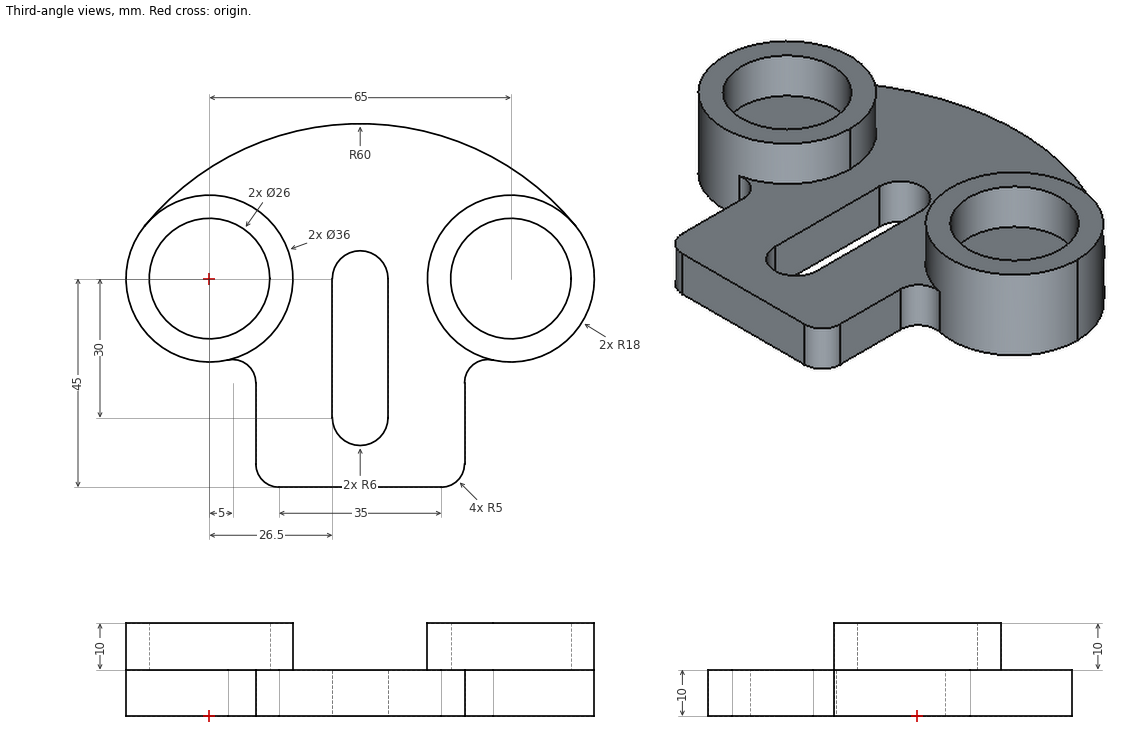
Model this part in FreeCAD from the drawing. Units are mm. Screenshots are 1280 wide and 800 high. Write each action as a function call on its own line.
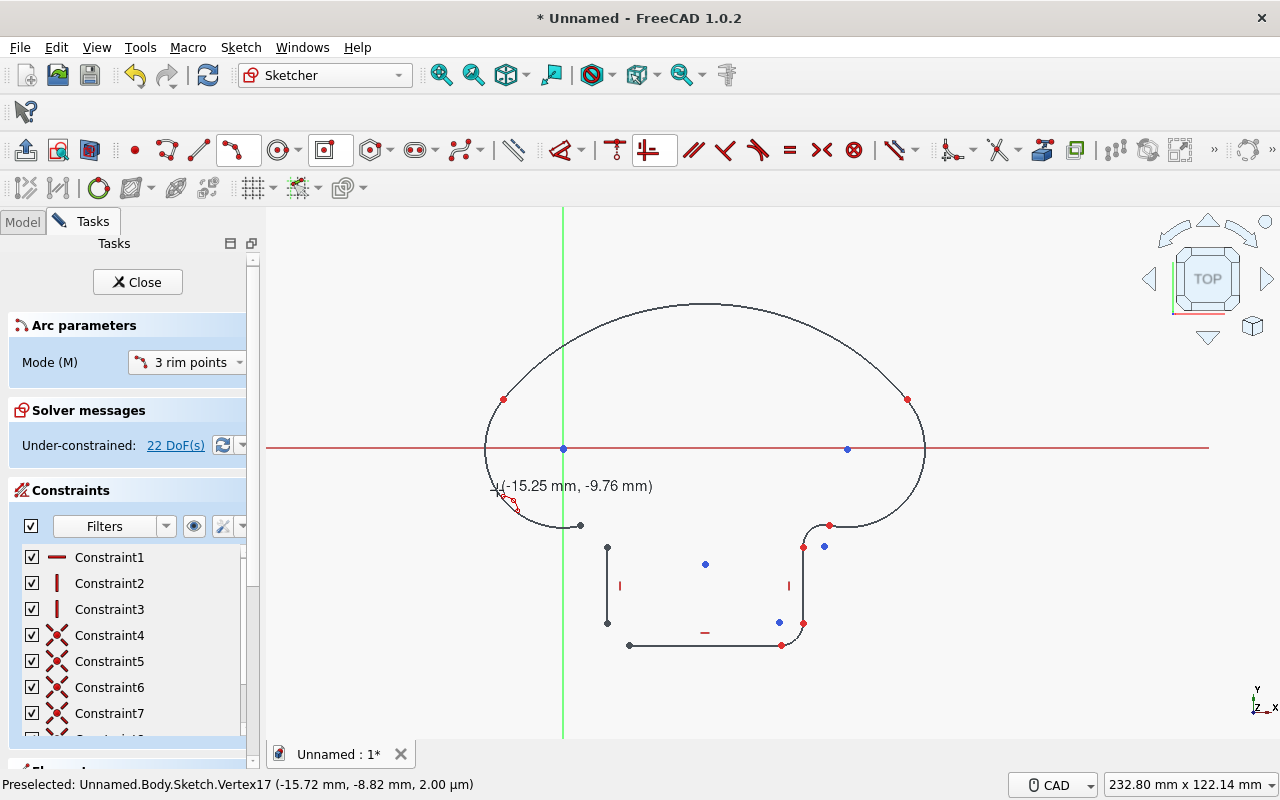
click(580, 526)
click(607, 548)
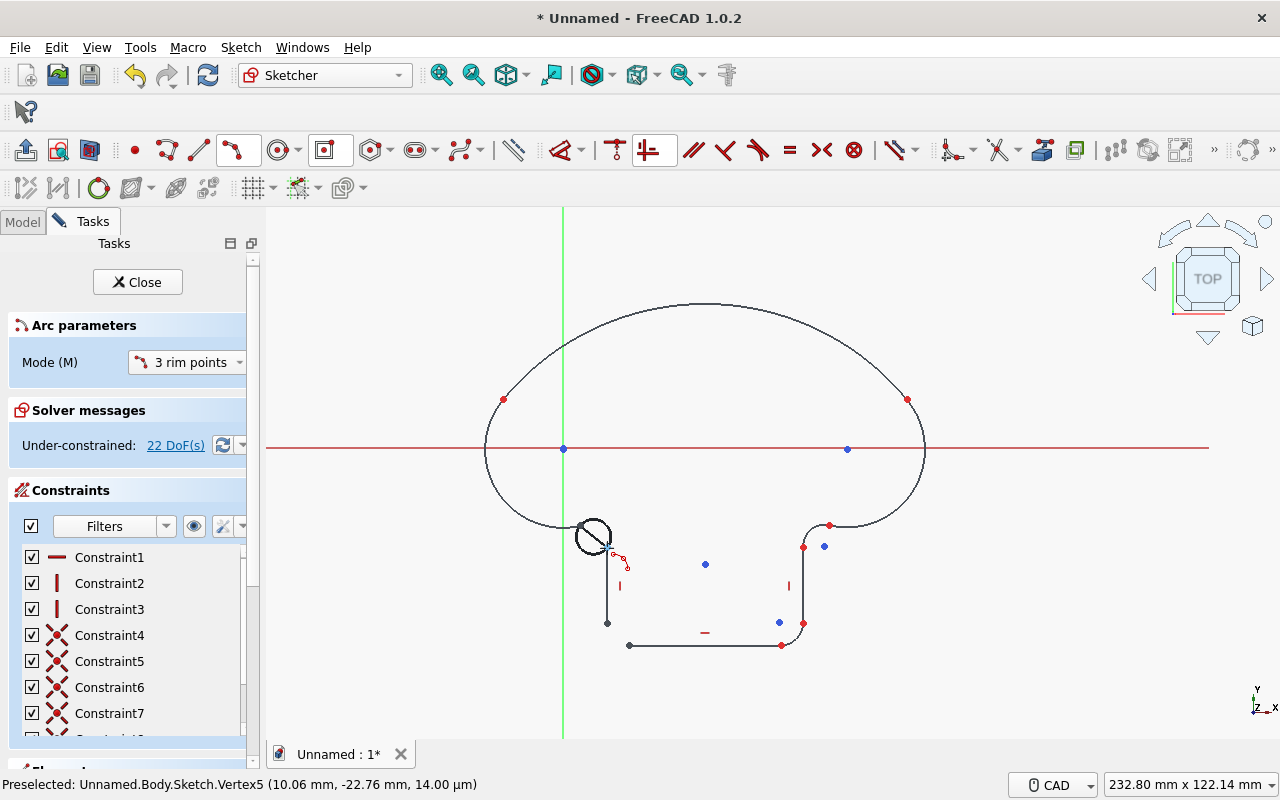
scroll(599, 529, up, 4)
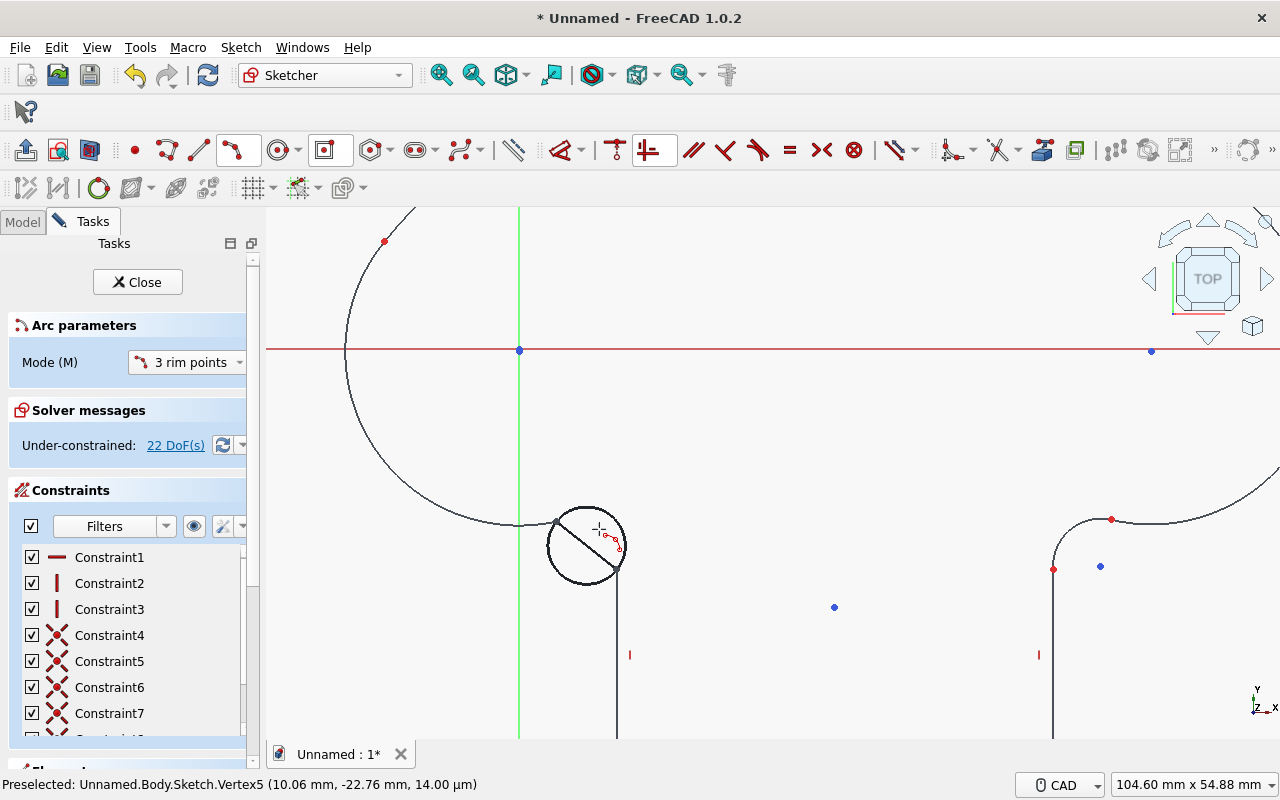
click(598, 529)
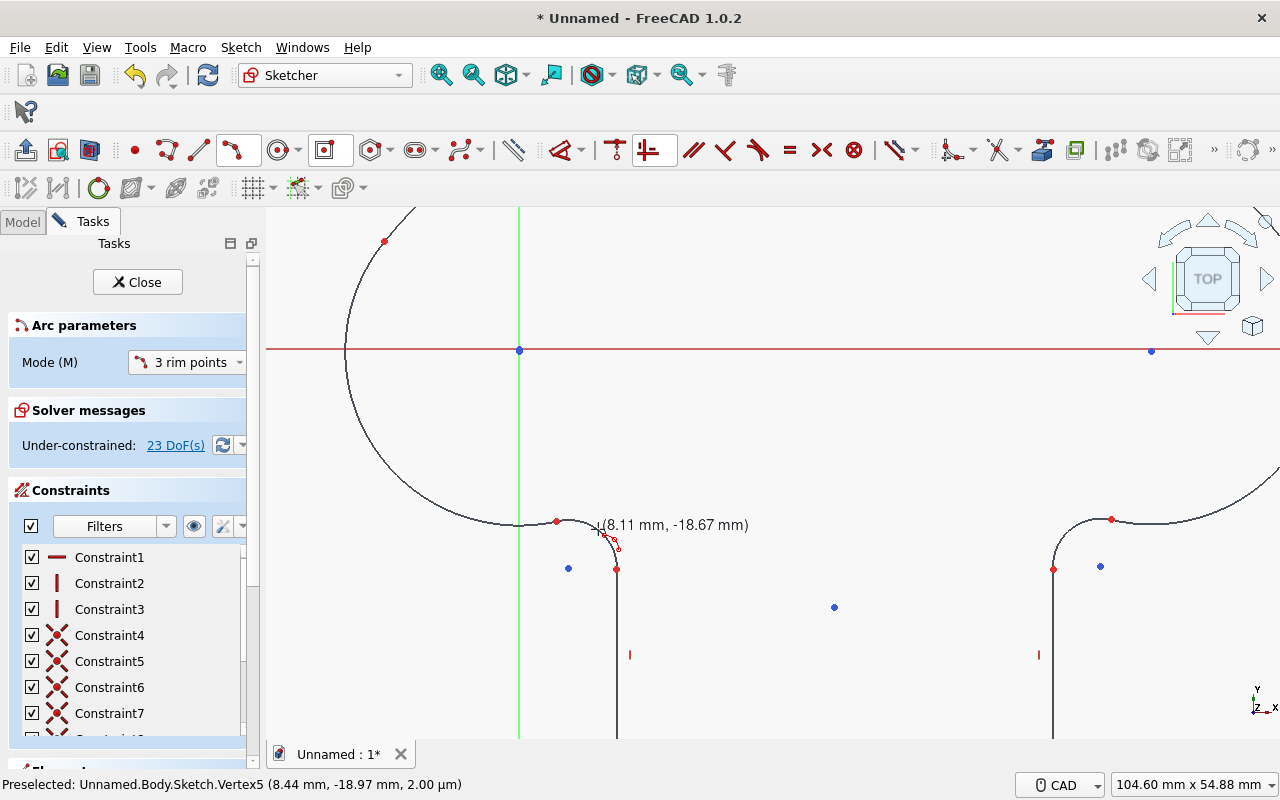
scroll(598, 528, down, 4)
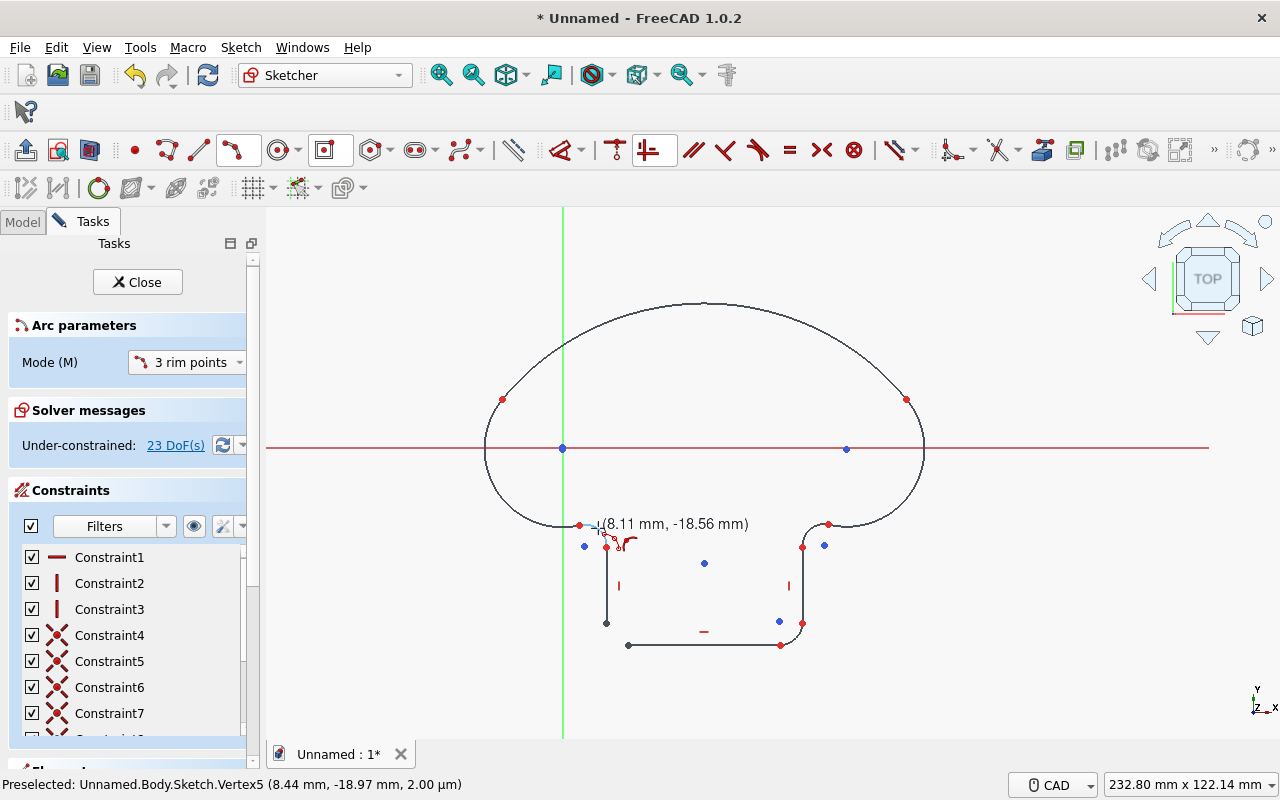
click(607, 623)
click(629, 645)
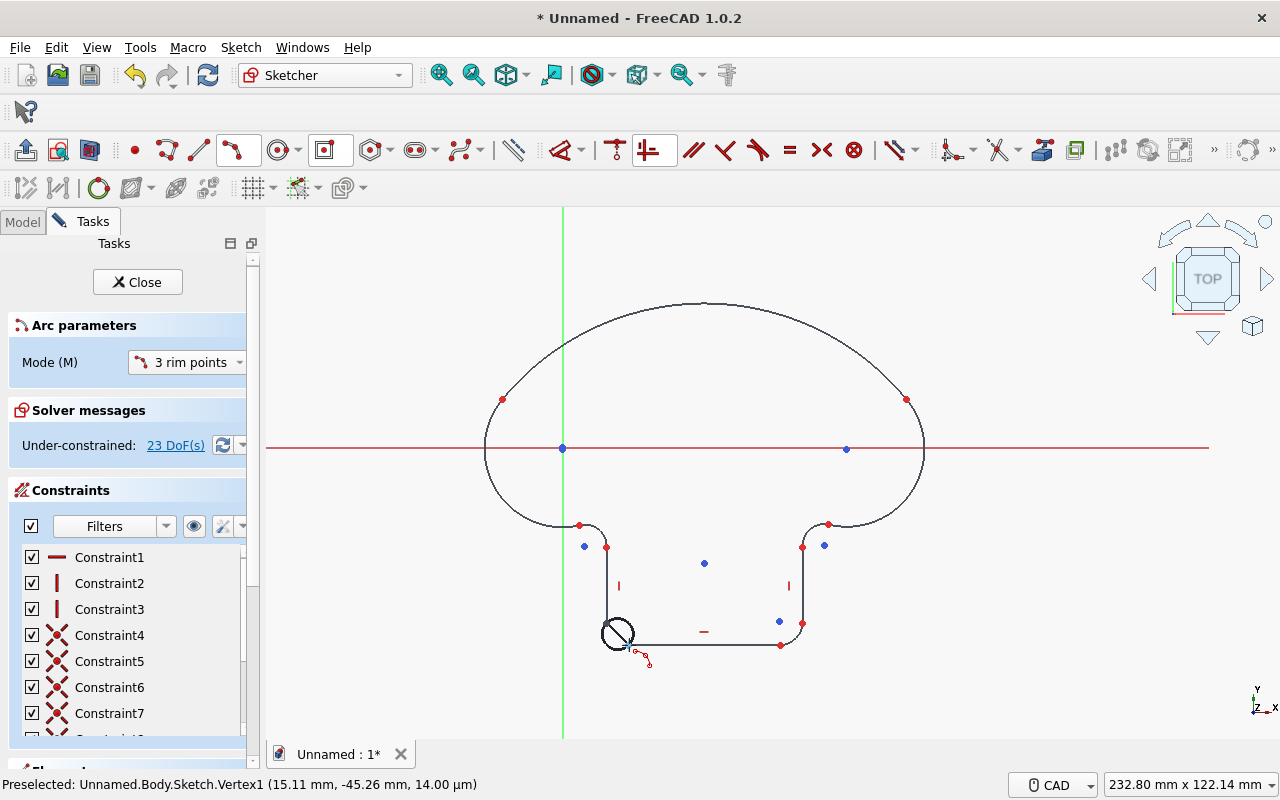
scroll(613, 638, up, 5)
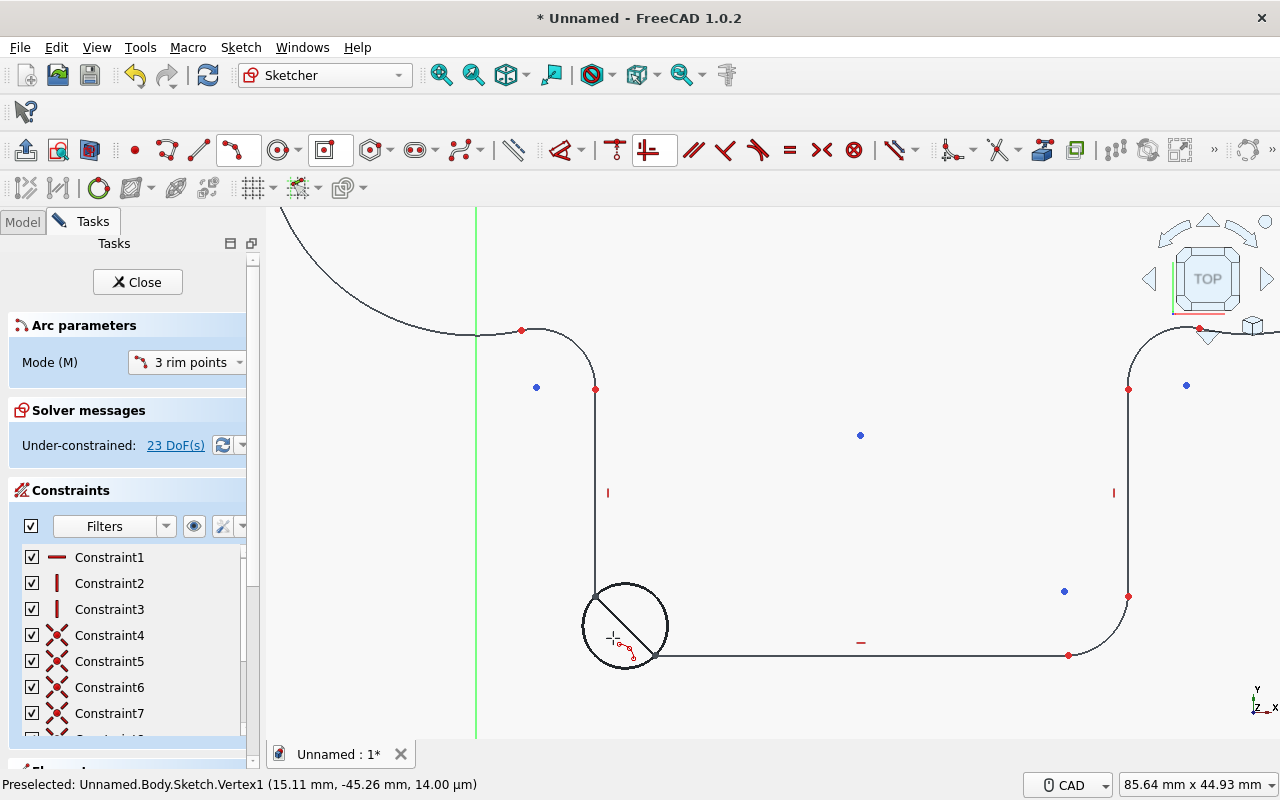
click(612, 635)
key(Escape)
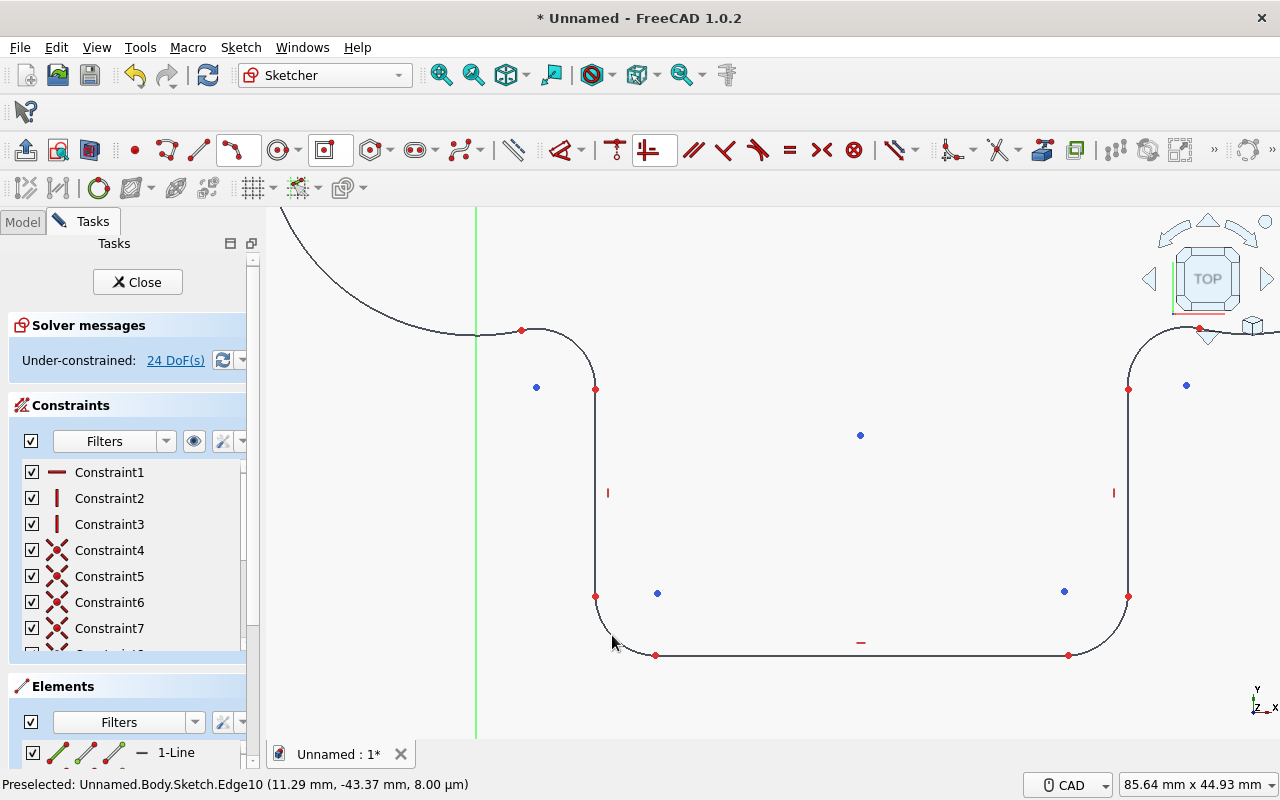
click(779, 656)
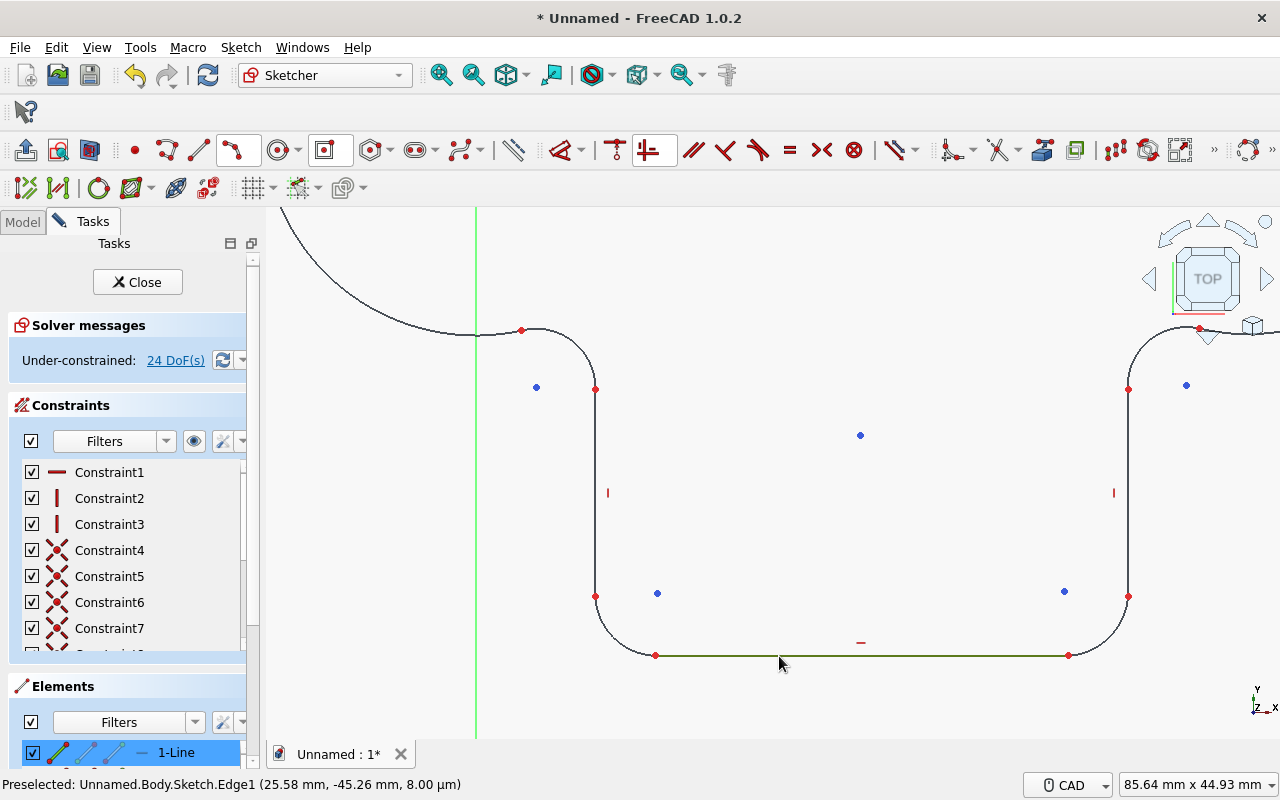
click(1095, 648)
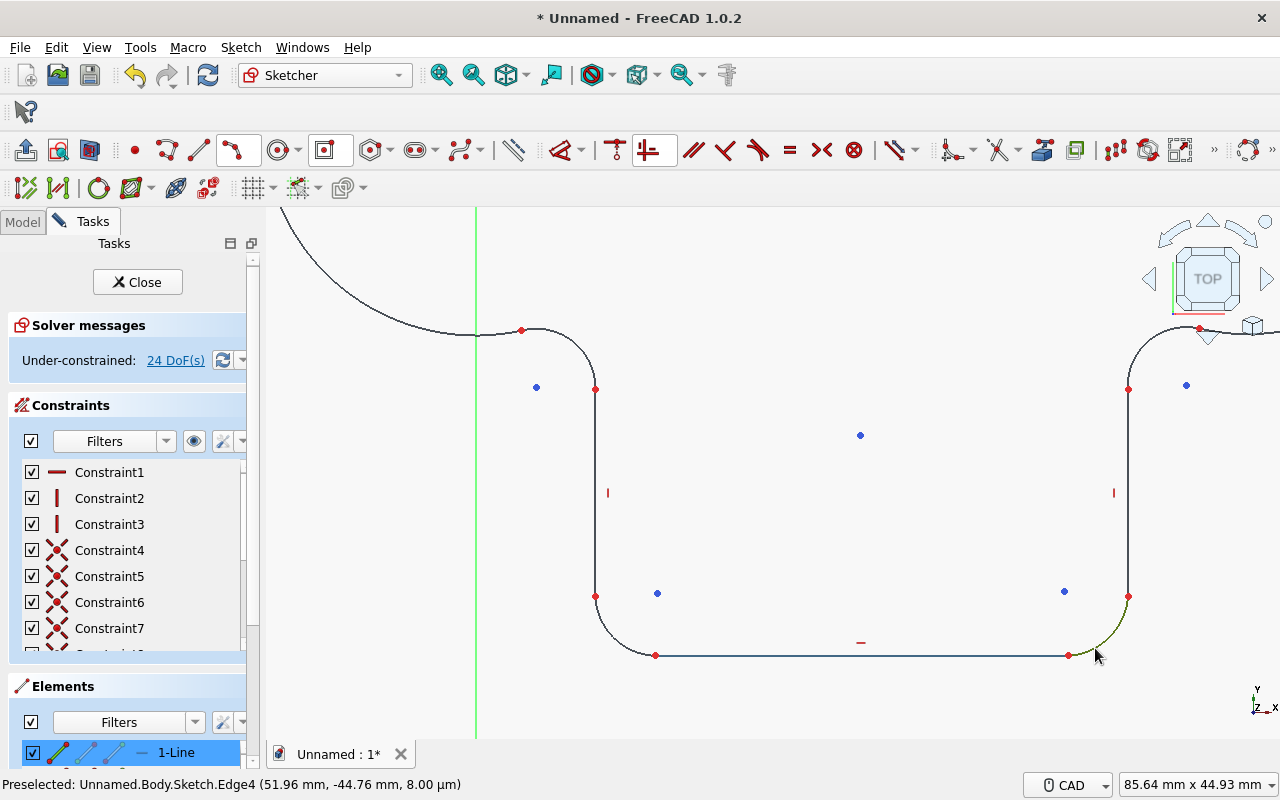
click(758, 150)